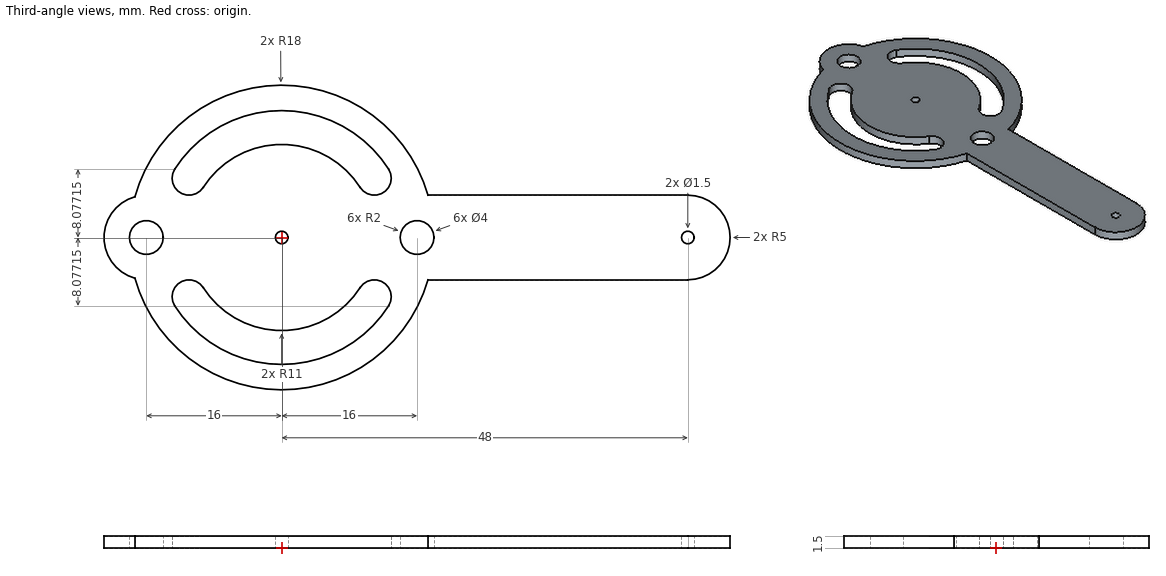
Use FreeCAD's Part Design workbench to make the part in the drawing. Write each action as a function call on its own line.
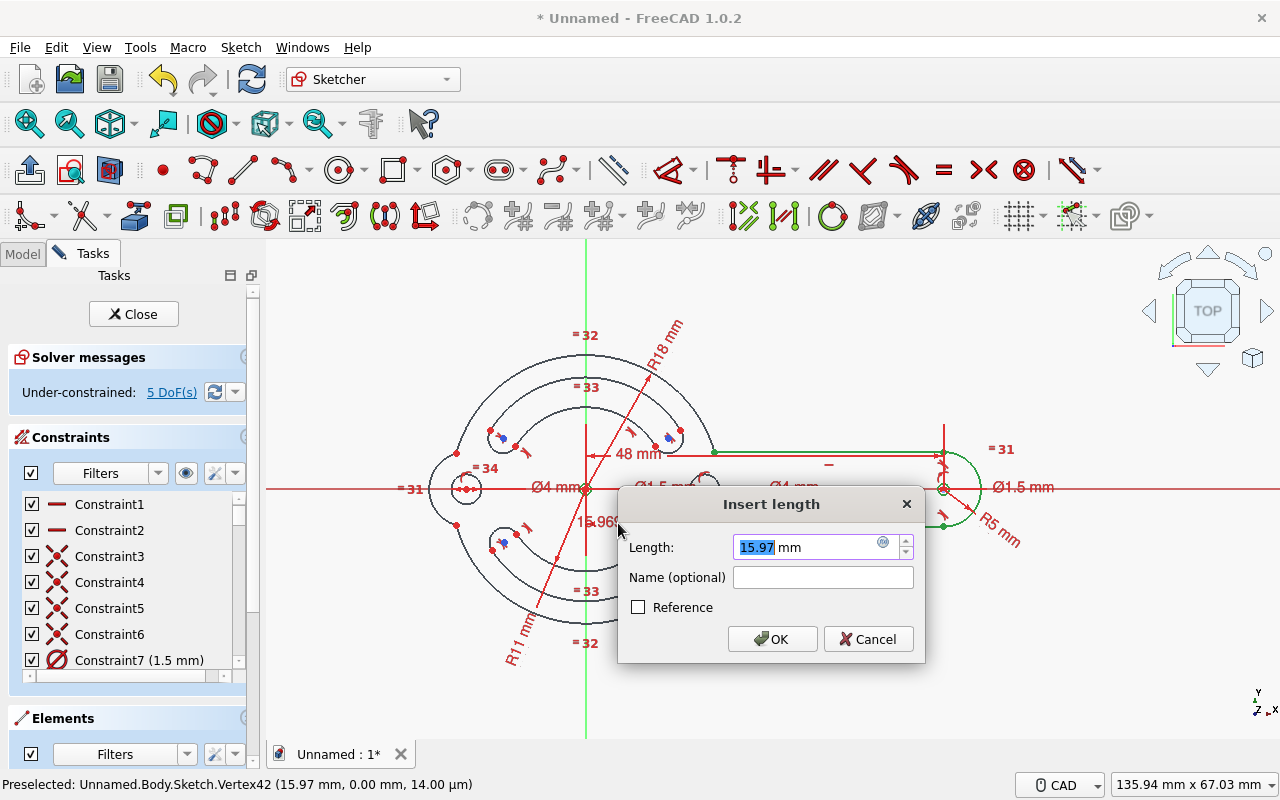
text(16)
key(Return)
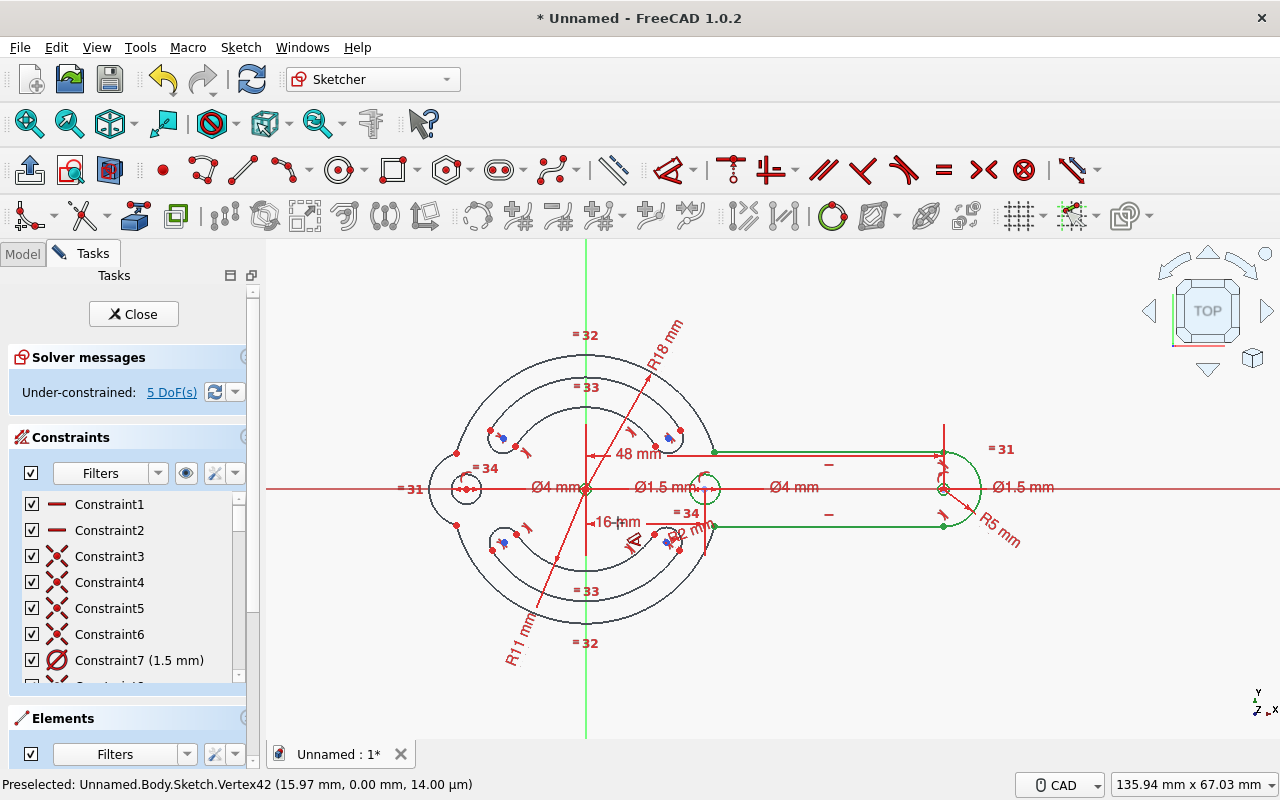
click(467, 489)
click(526, 523)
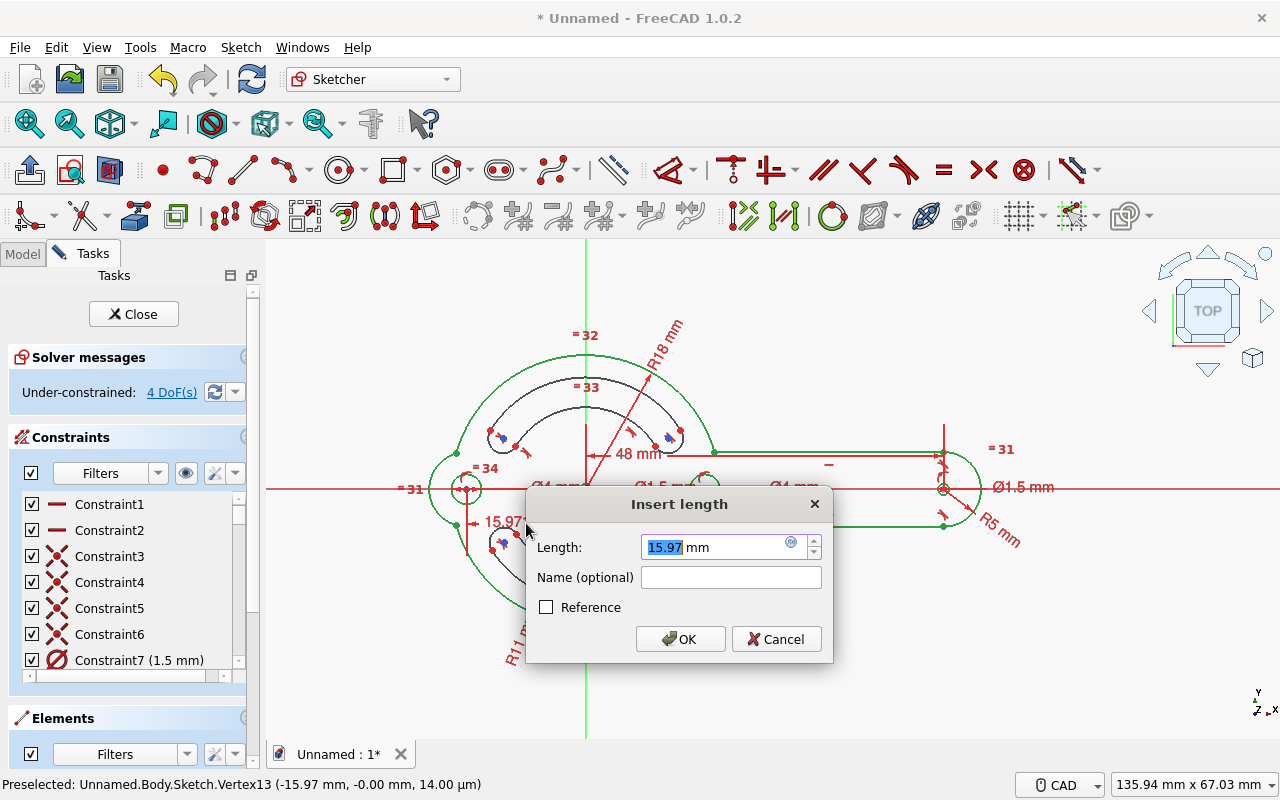
text(16)
key(Return)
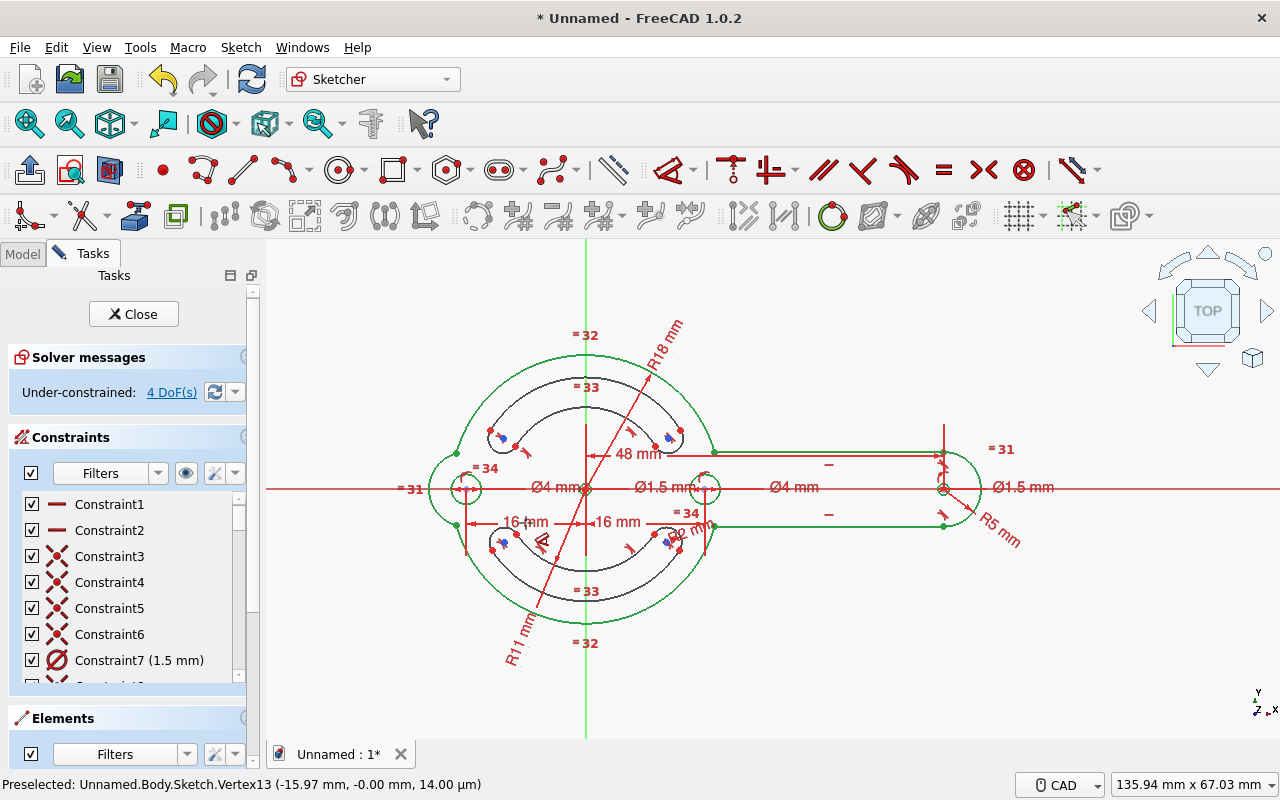
click(679, 551)
click(737, 506)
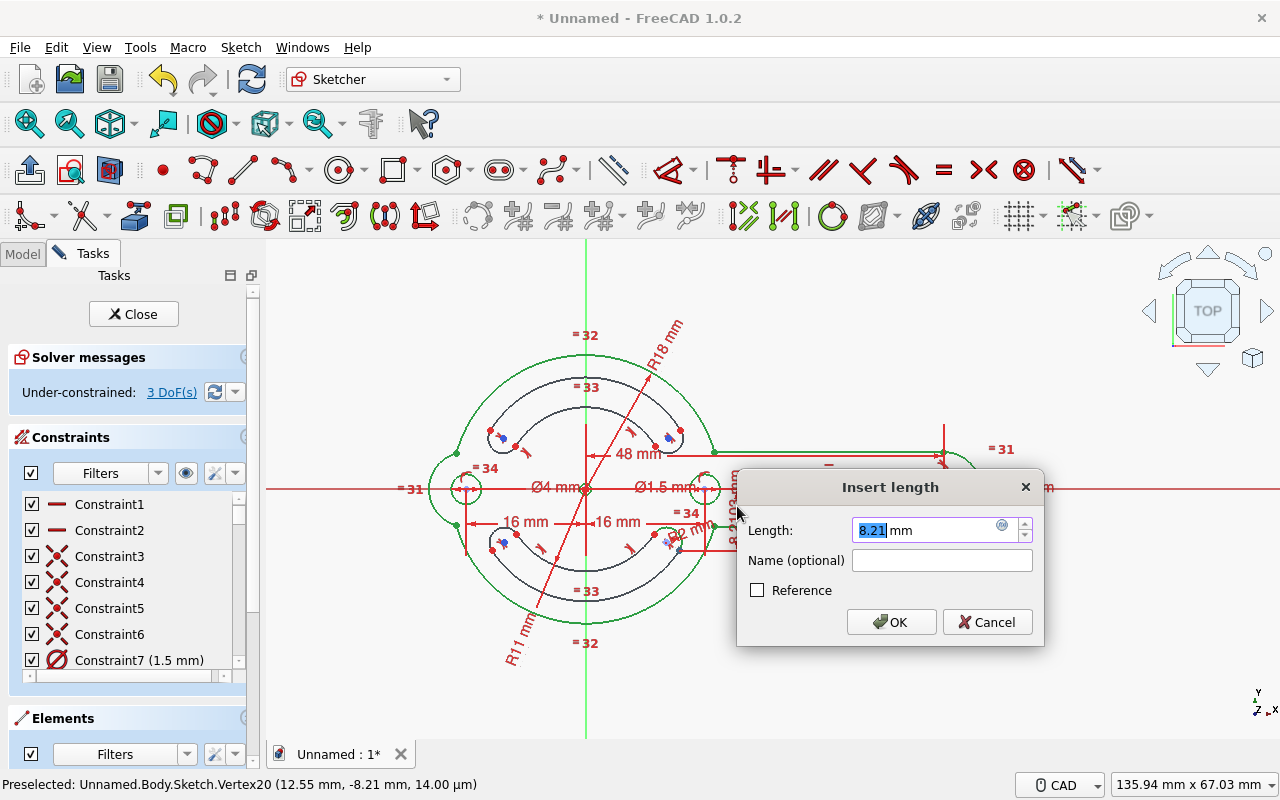
text(8.07715)
key(Return)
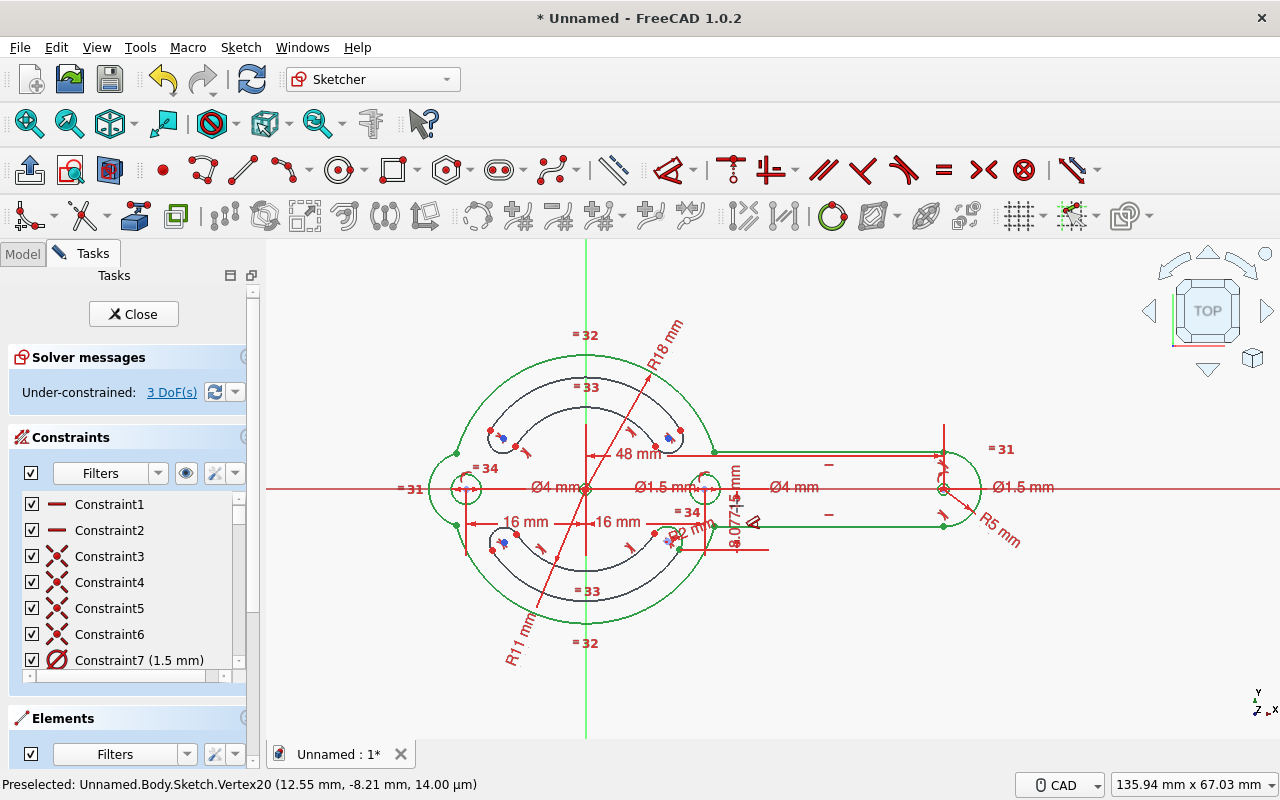
click(492, 551)
click(434, 534)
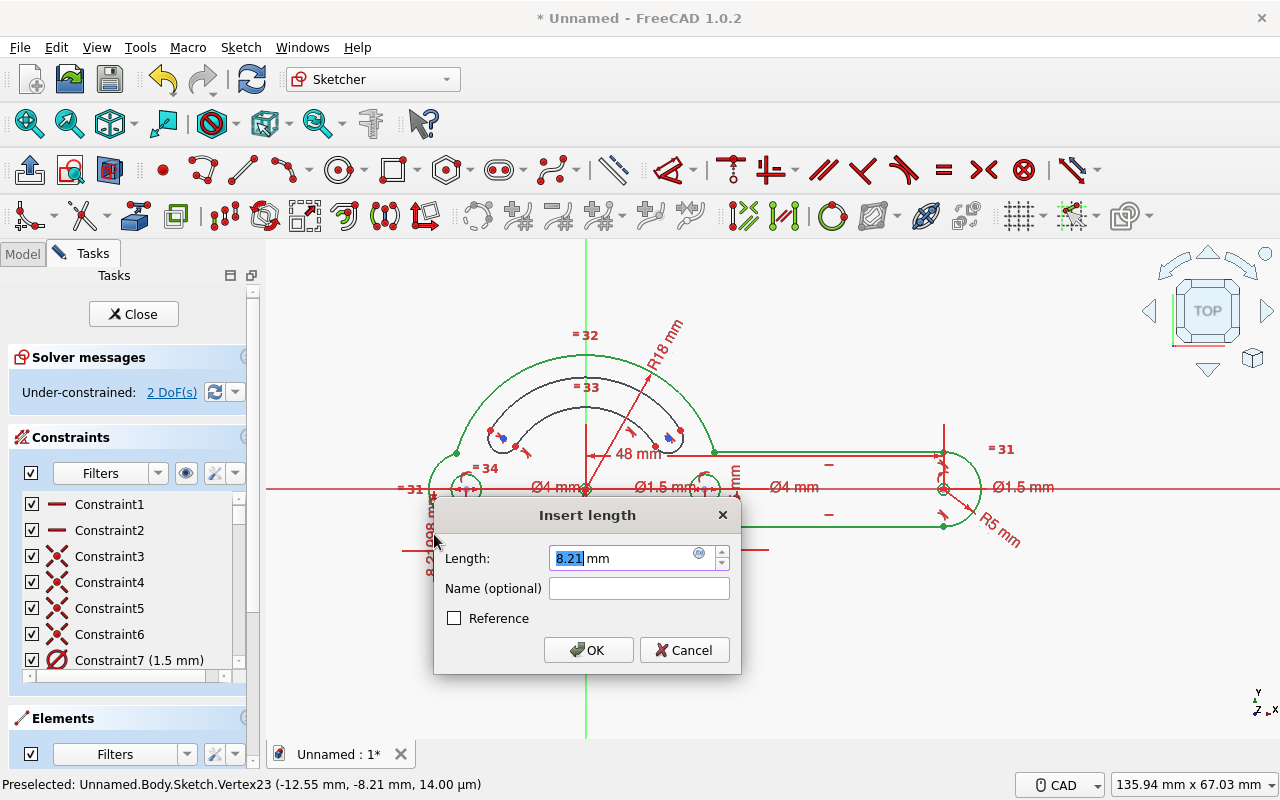
text(8.07715)
key(Return)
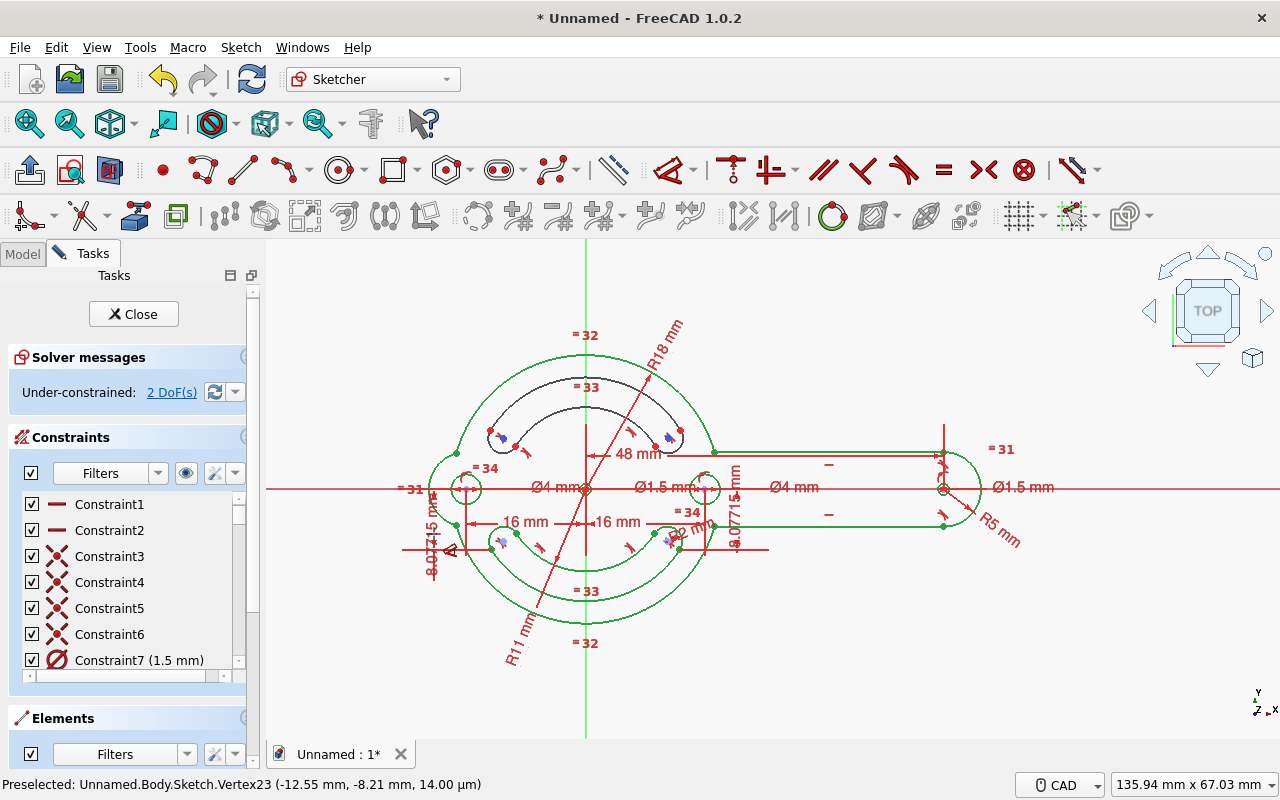
click(490, 431)
click(432, 446)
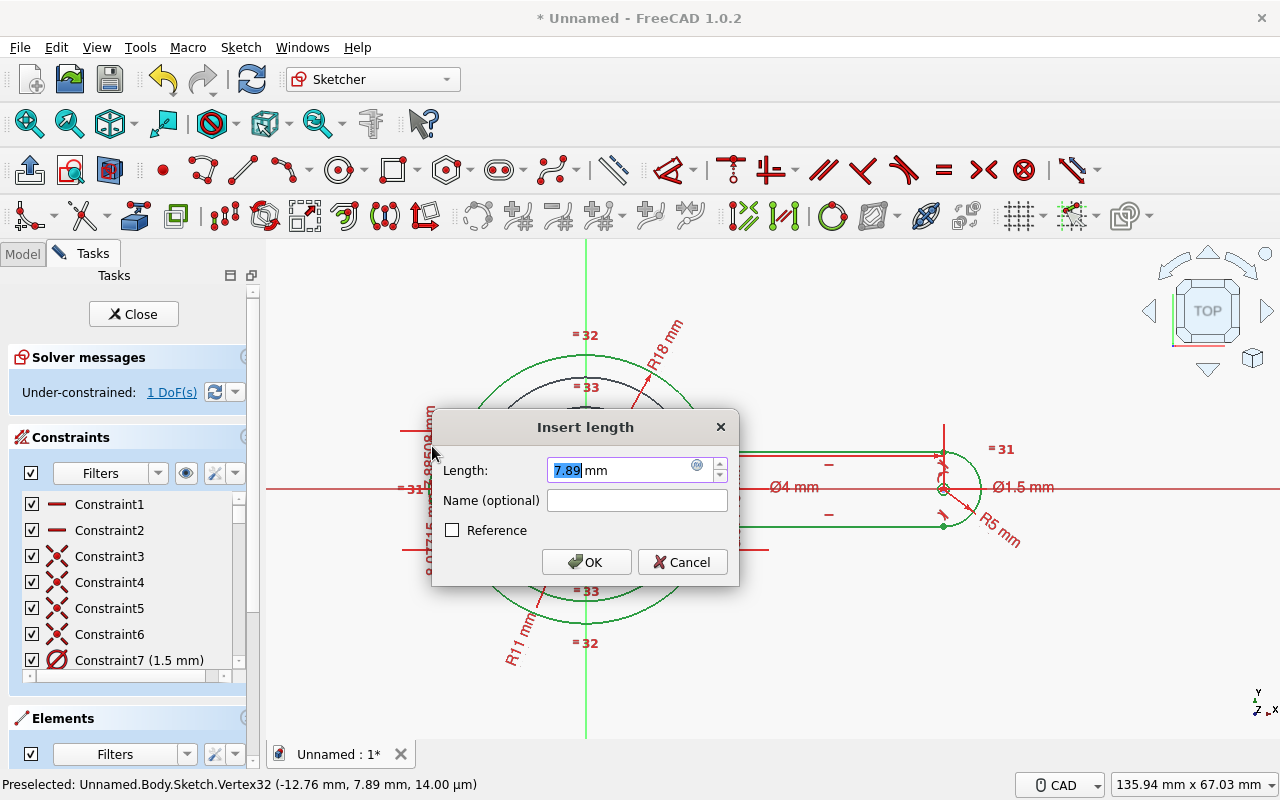
text(8.07715)
key(Return)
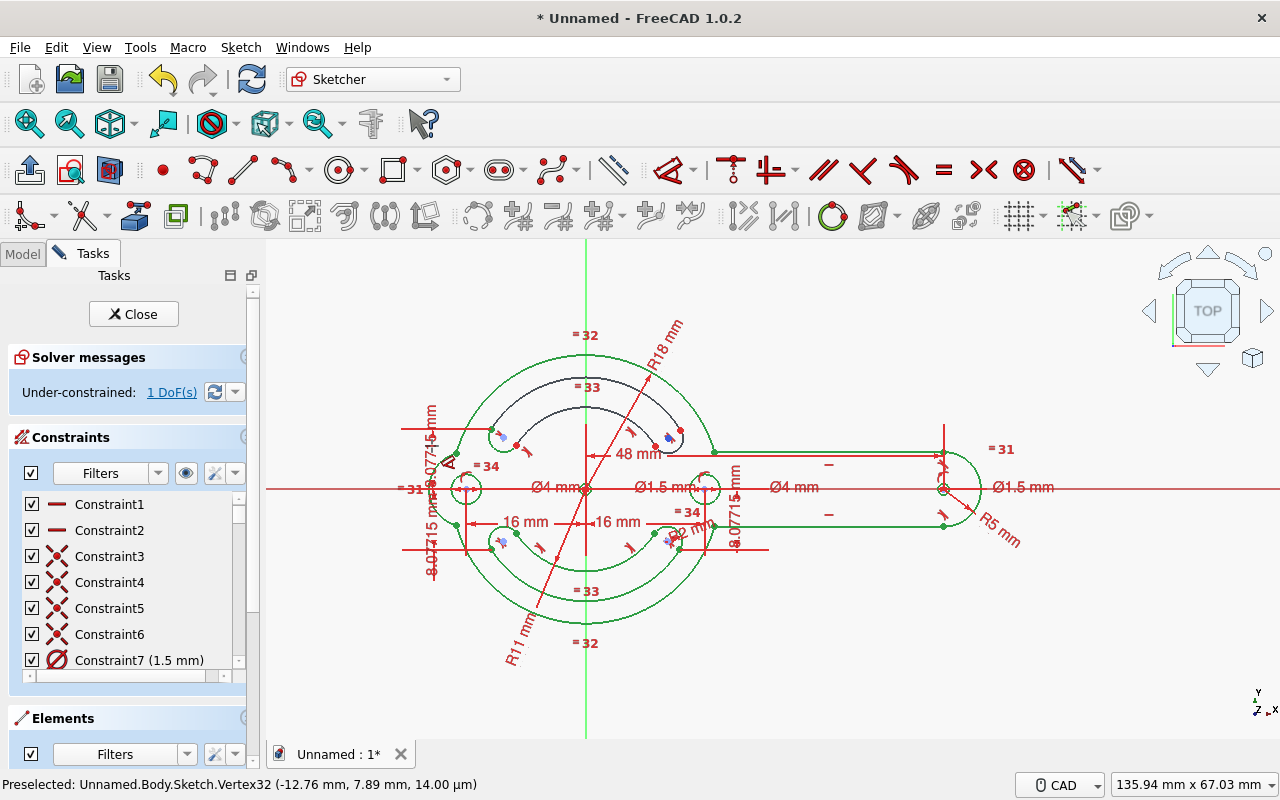
click(681, 431)
click(552, 460)